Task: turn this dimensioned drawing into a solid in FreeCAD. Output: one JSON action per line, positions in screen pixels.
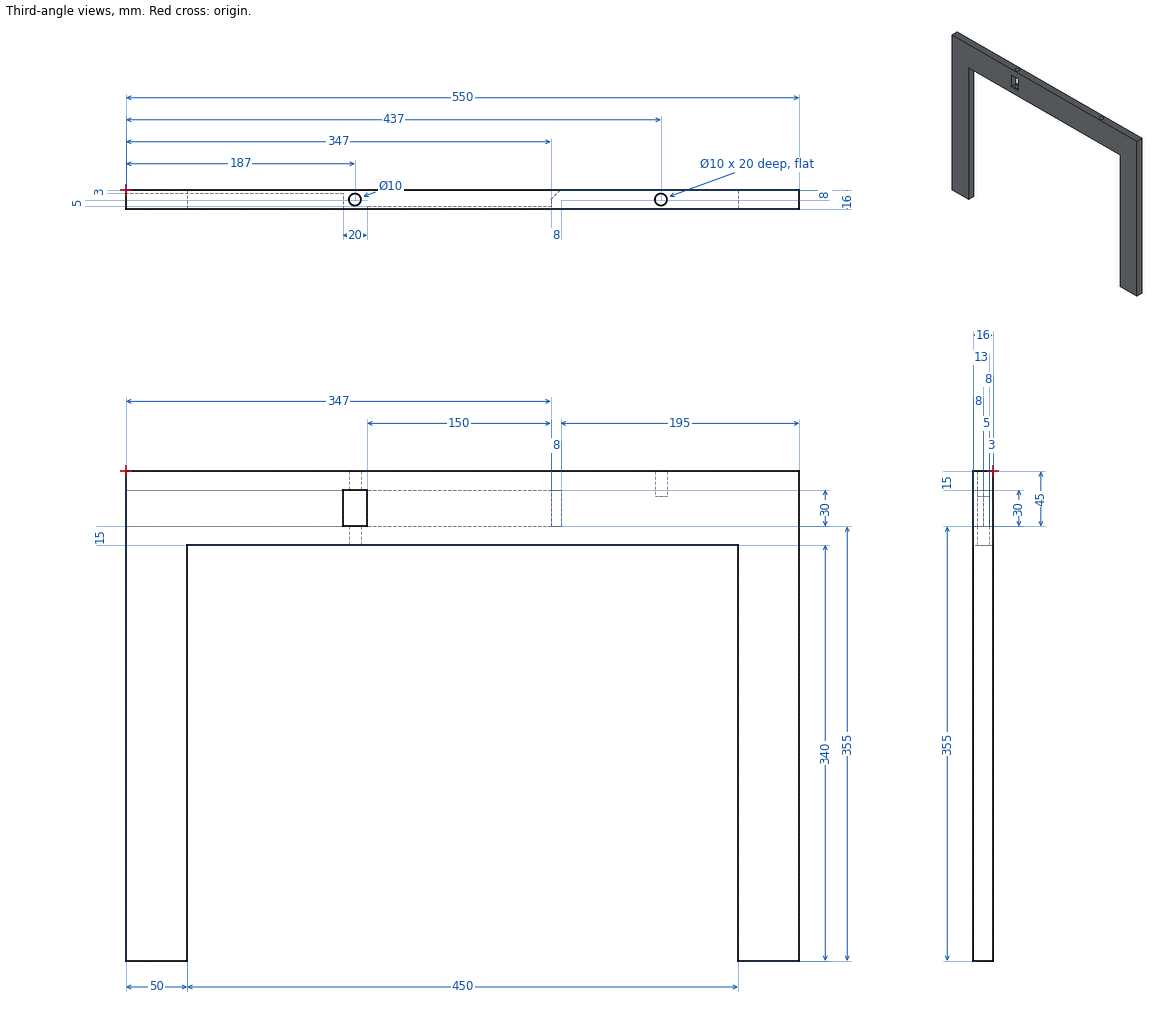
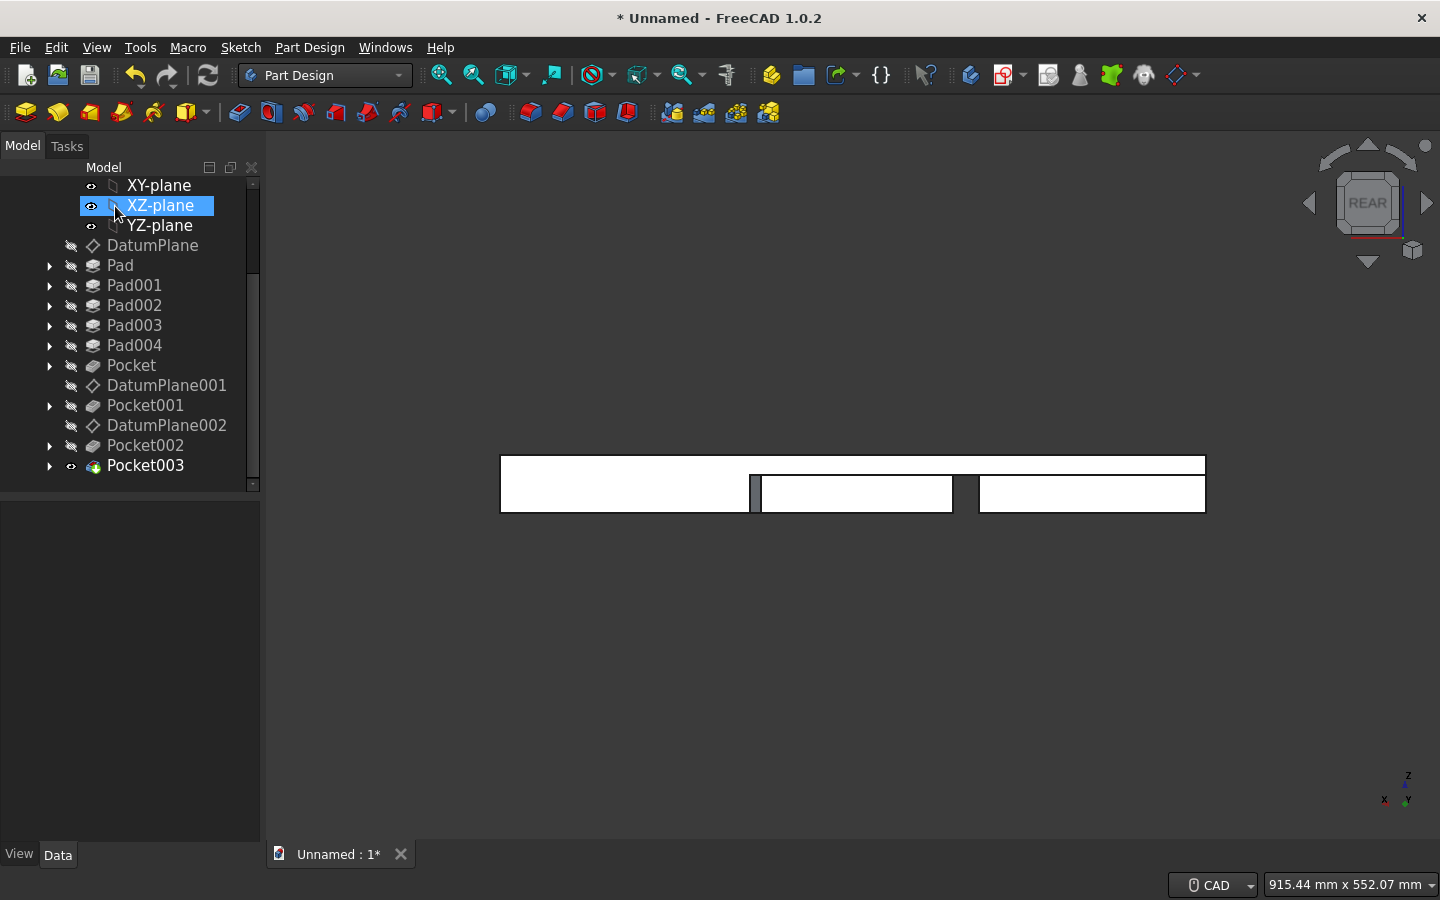
{"action": "key", "text": "5"}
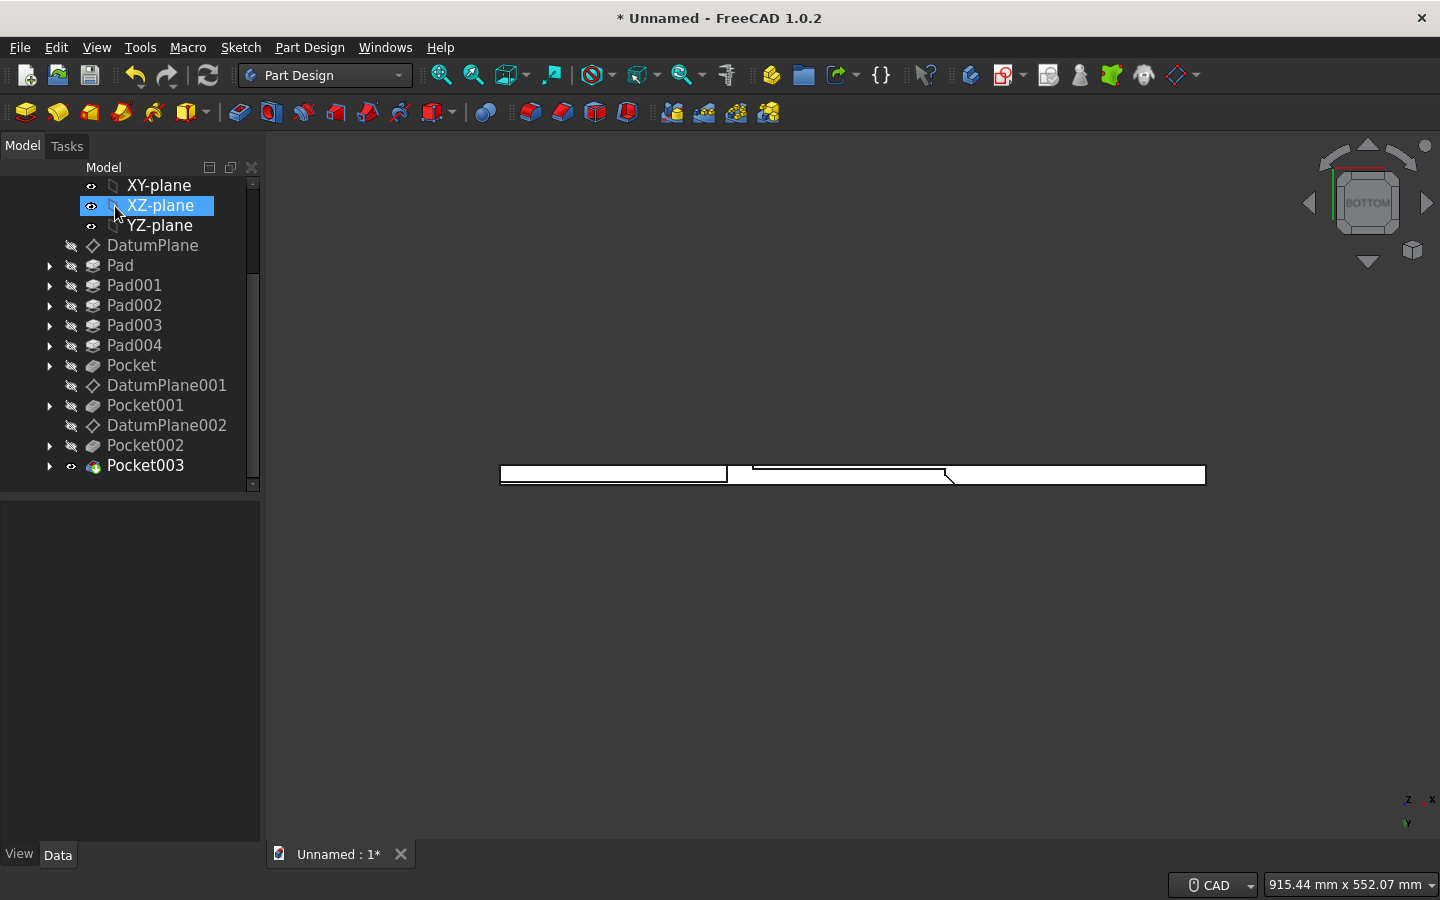
{"action": "left_click", "coordinate": [1173, 474]}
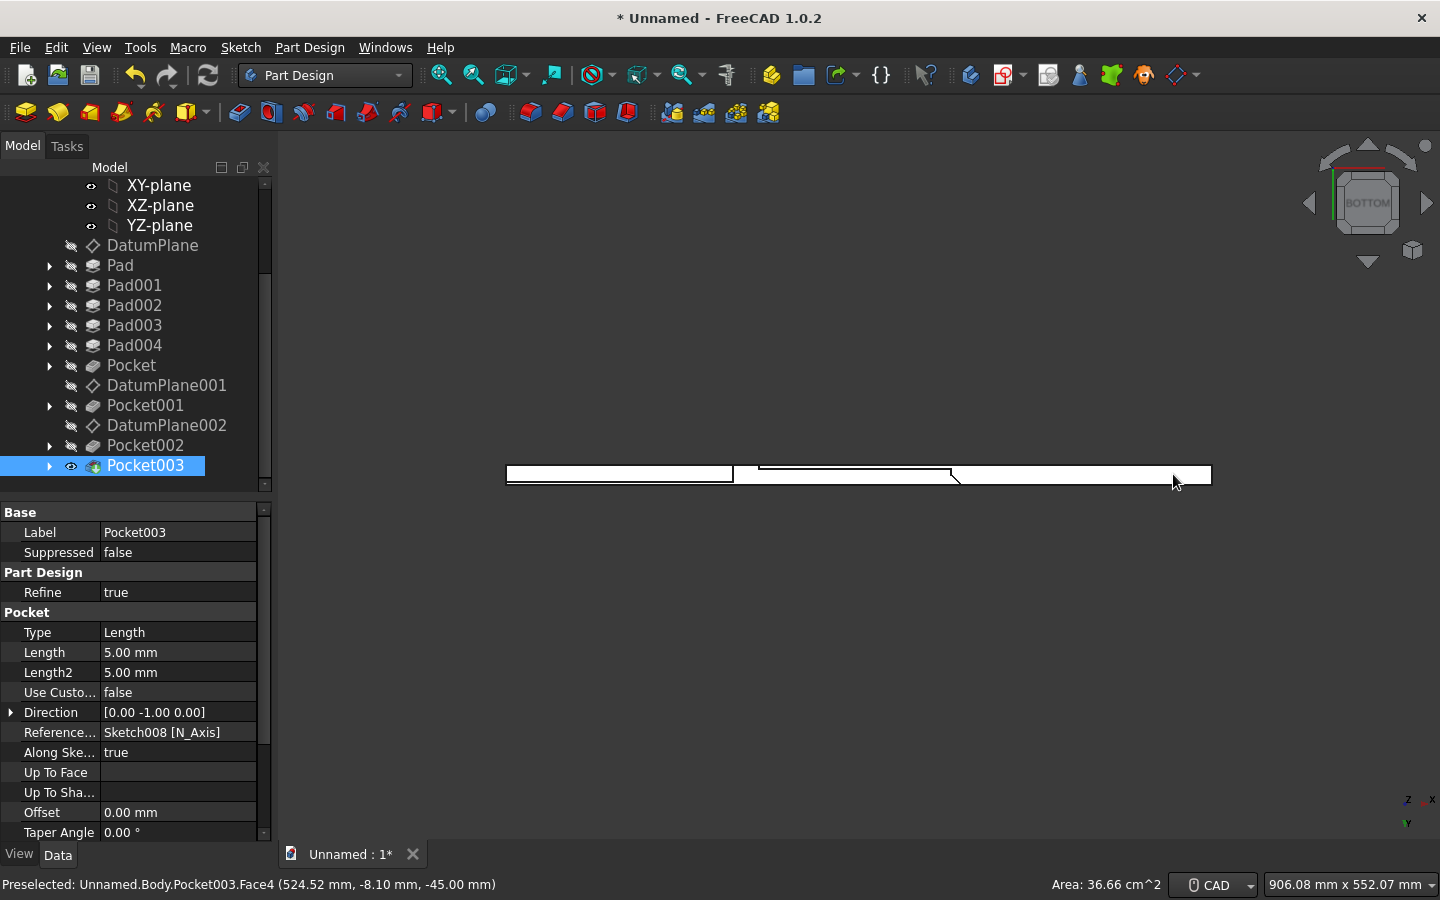
{"action": "left_click", "coordinate": [1004, 76]}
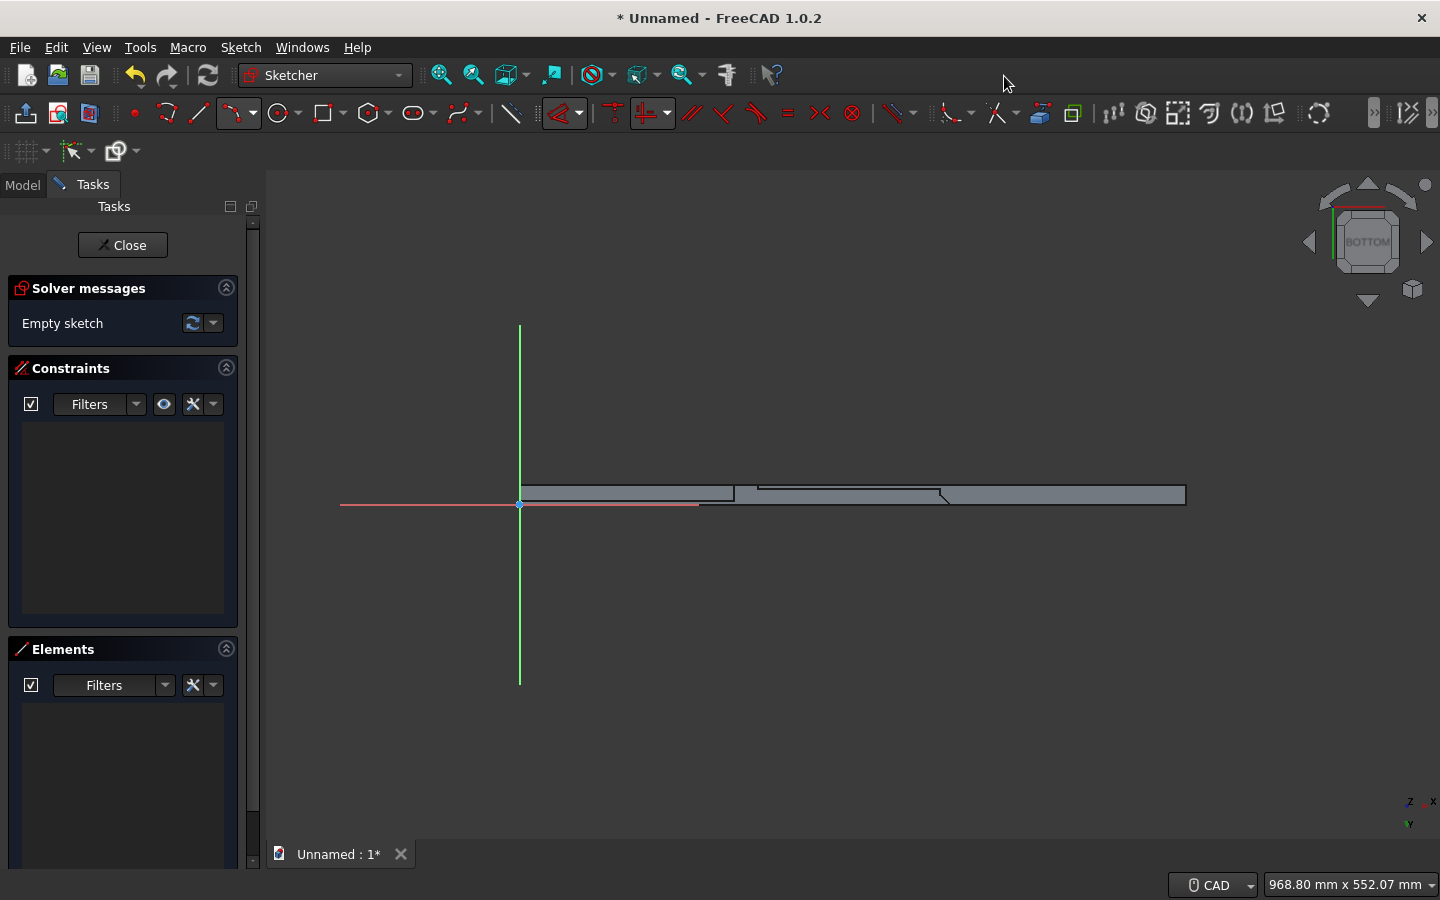
{"action": "left_click", "coordinate": [324, 114]}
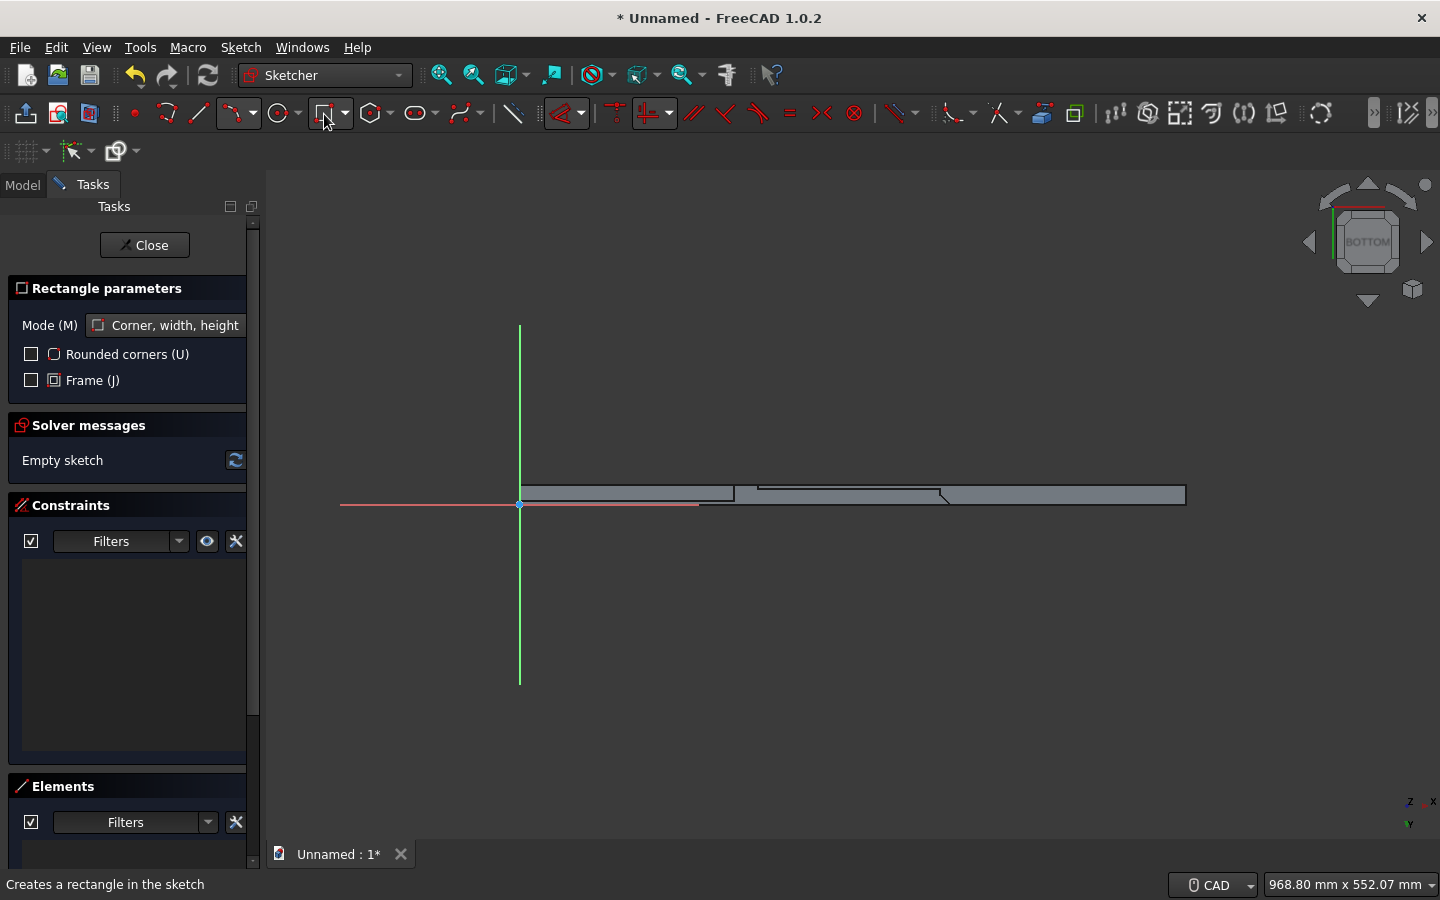
{"action": "left_click", "coordinate": [520, 505]}
{"action": "left_click", "coordinate": [1186, 485]}
{"action": "key", "text": "Escape"}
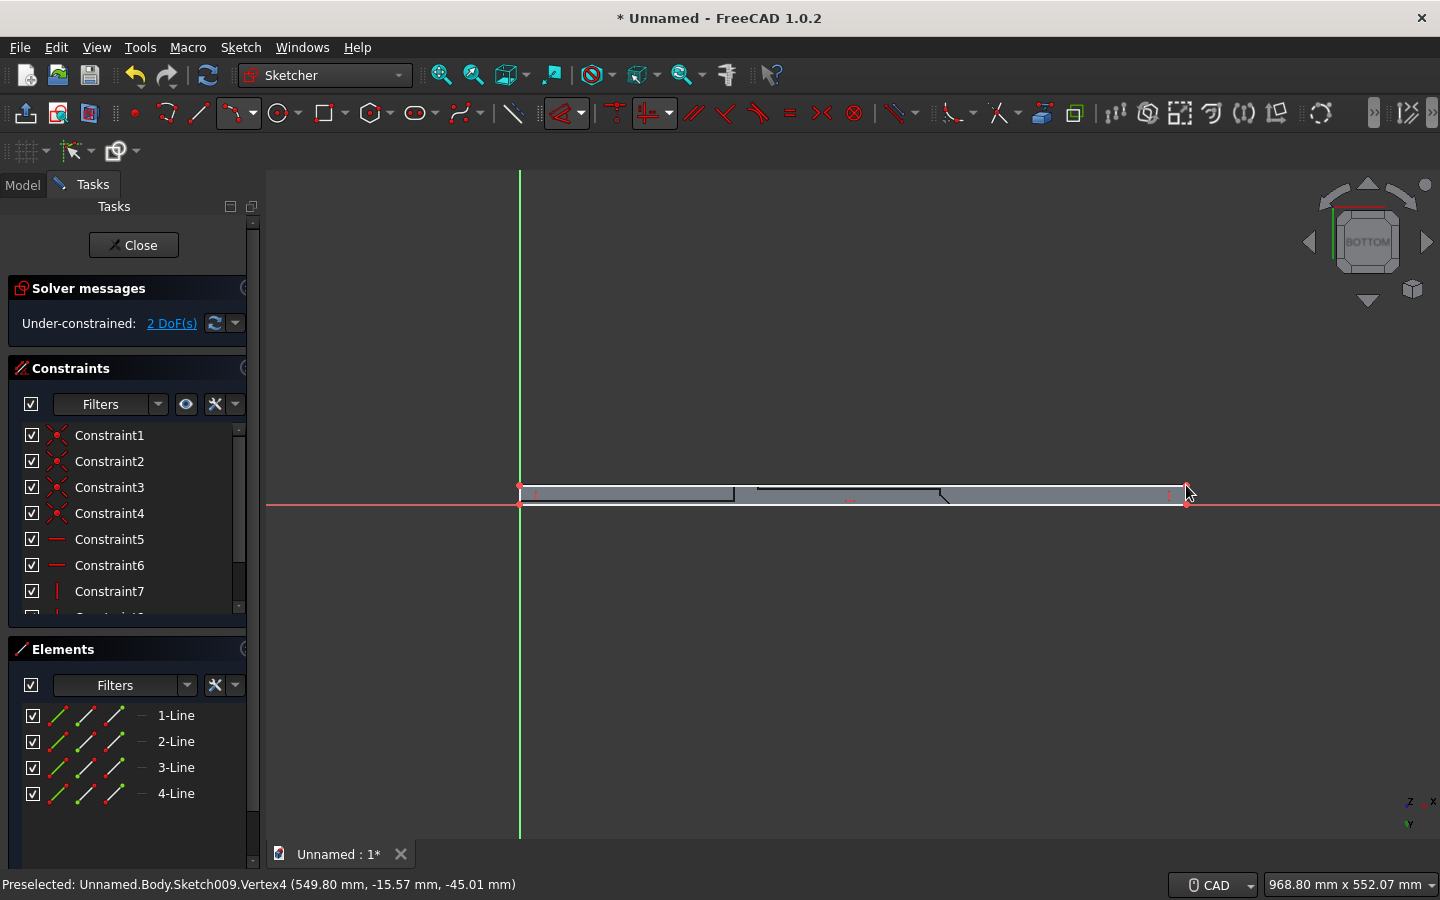
{"action": "scroll", "coordinate": [1186, 495], "scroll_direction": "up", "scroll_amount": 4}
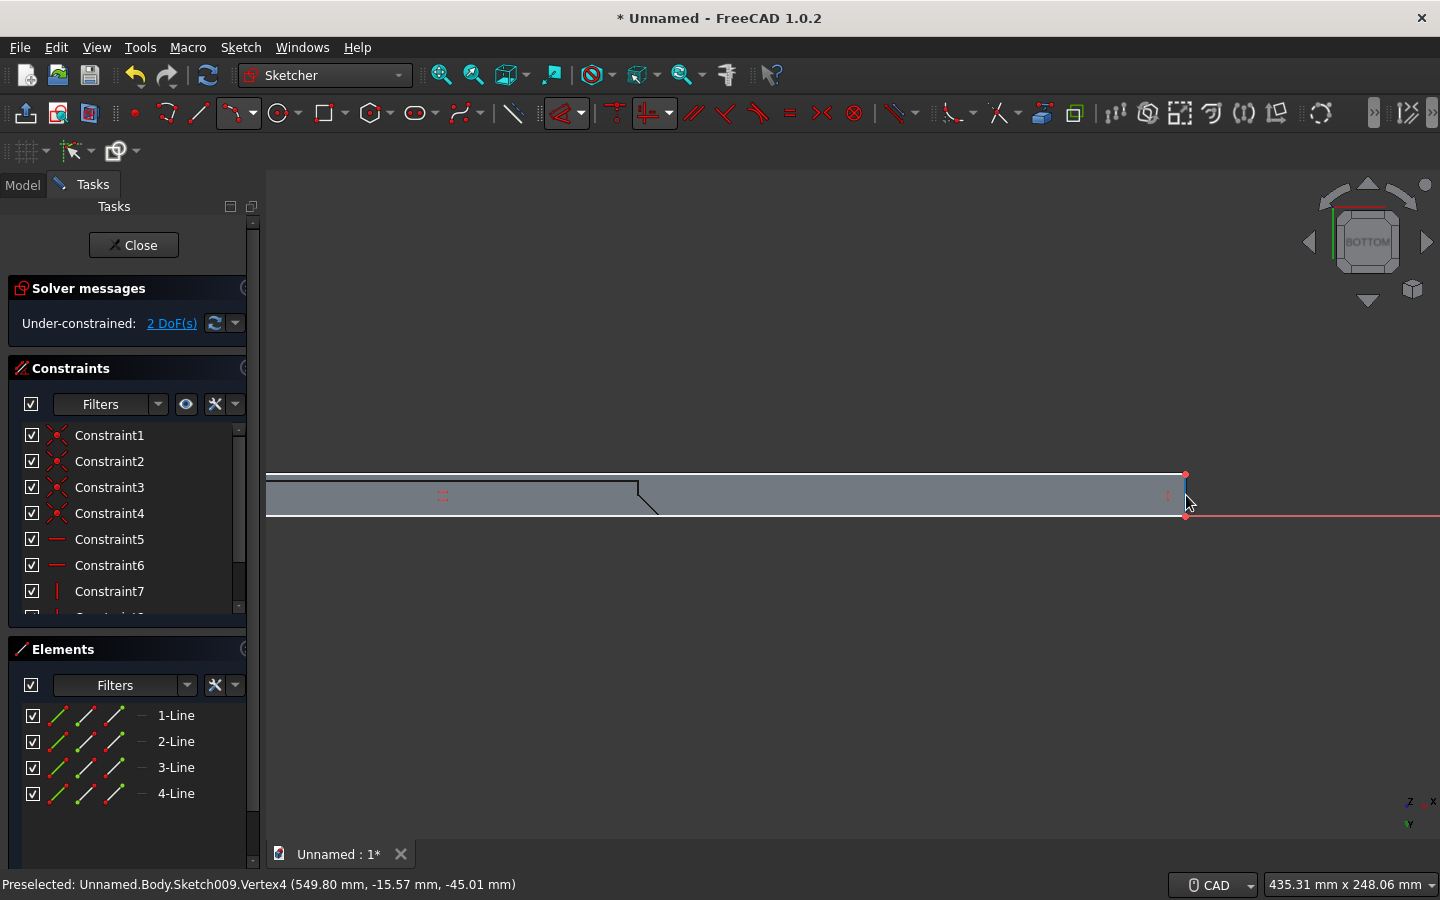
{"action": "left_click", "coordinate": [1185, 495]}